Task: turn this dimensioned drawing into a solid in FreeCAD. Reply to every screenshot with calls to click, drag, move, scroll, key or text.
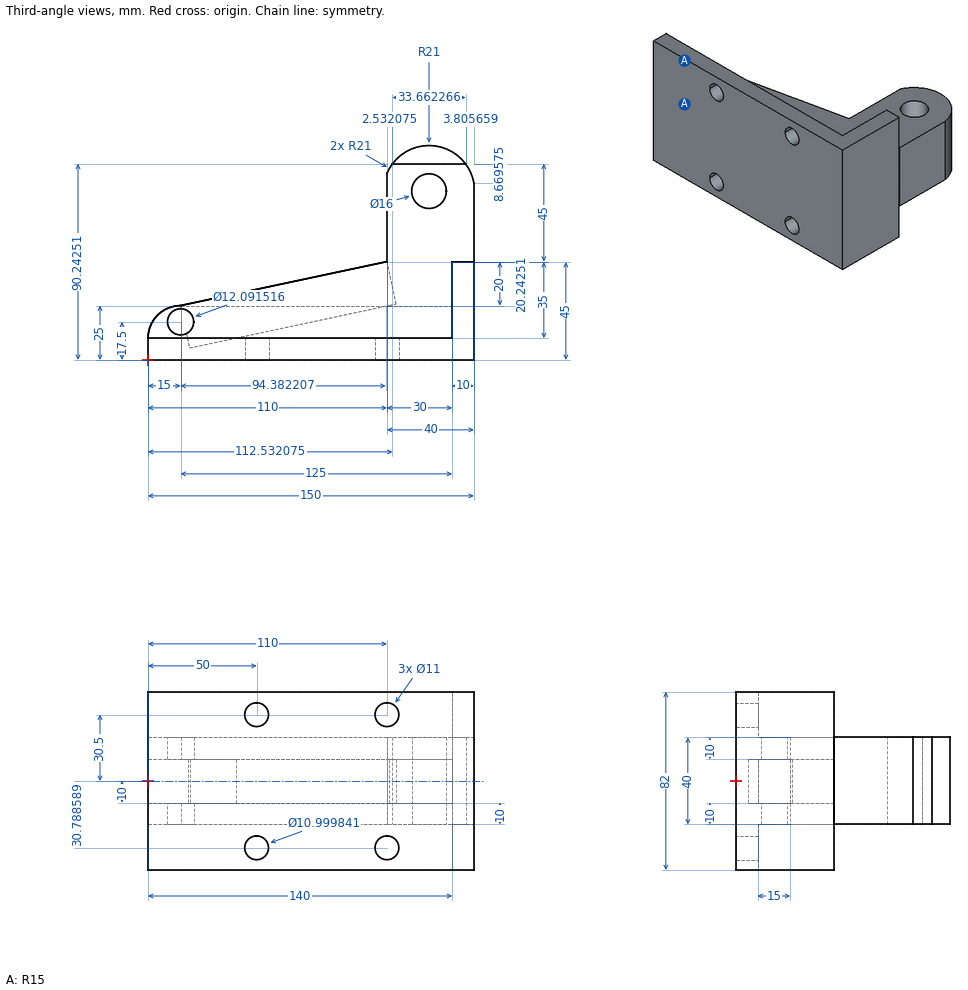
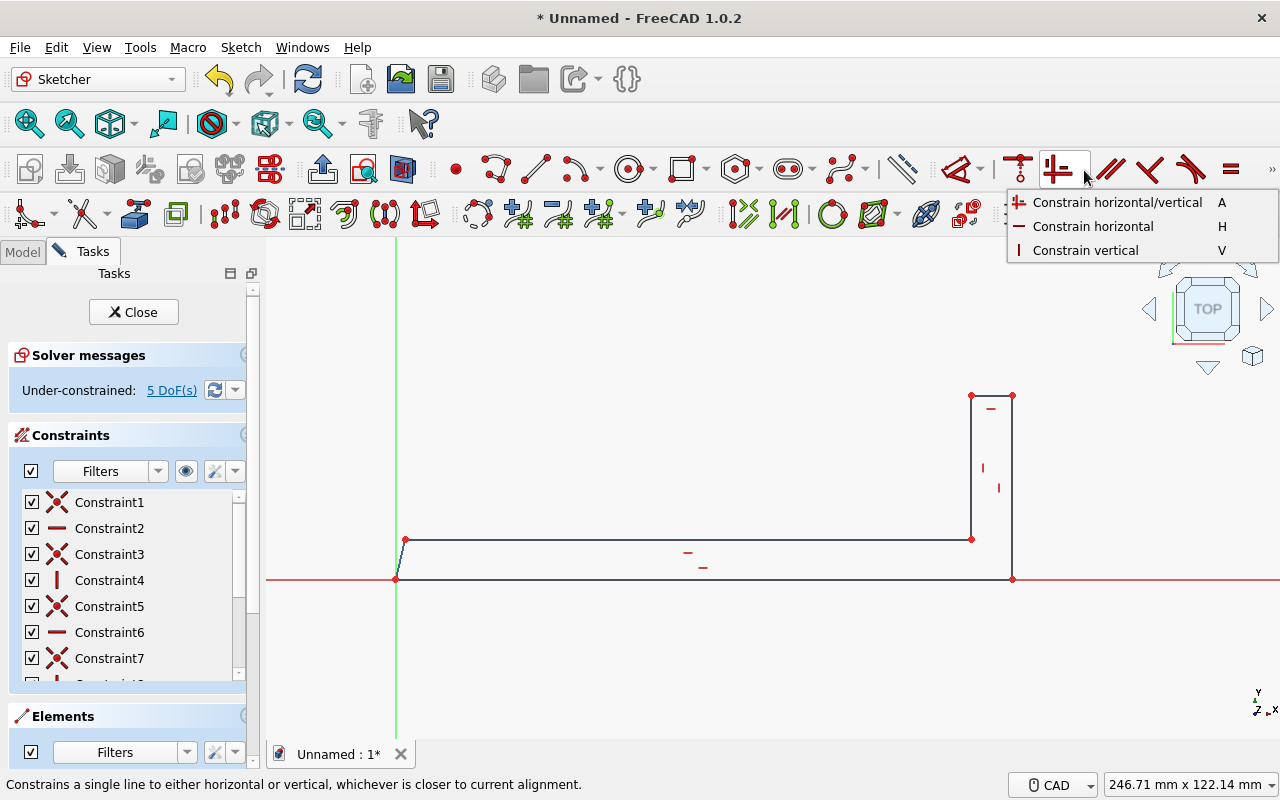
click(1143, 250)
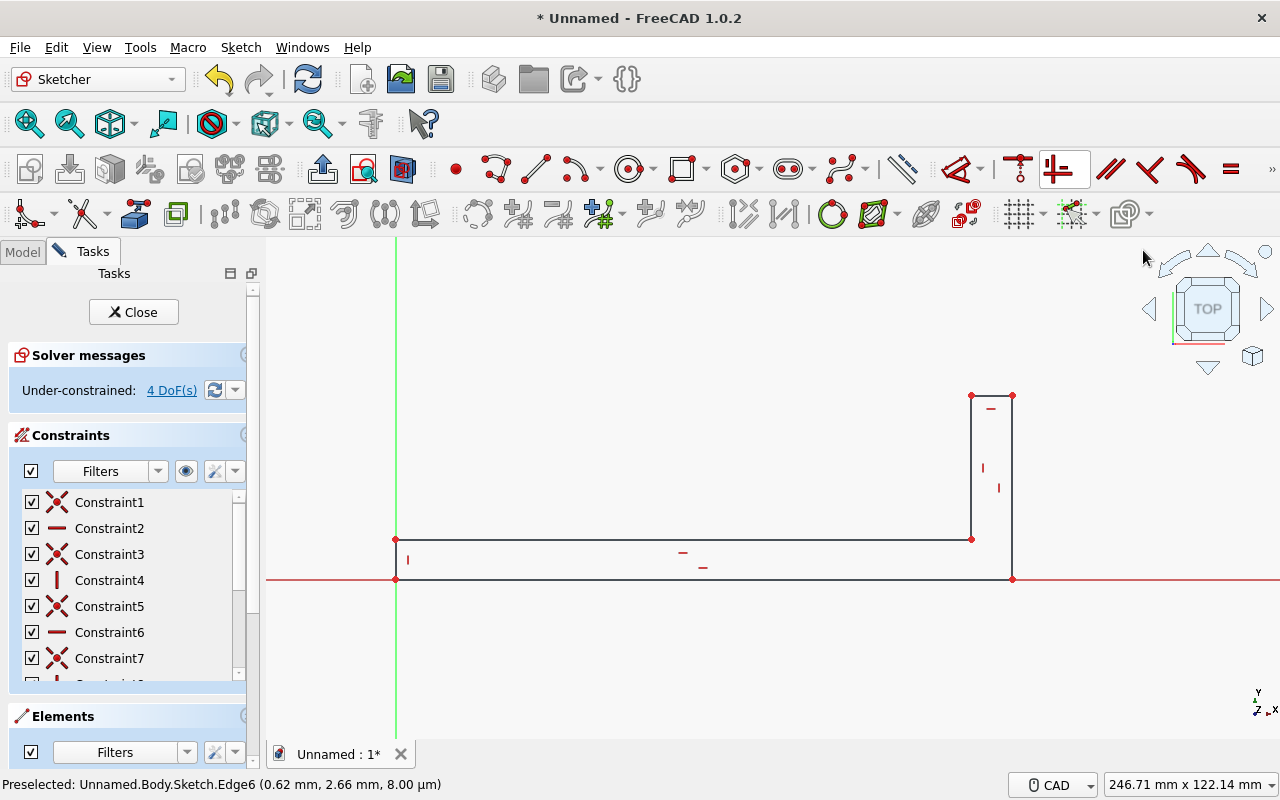
key(d)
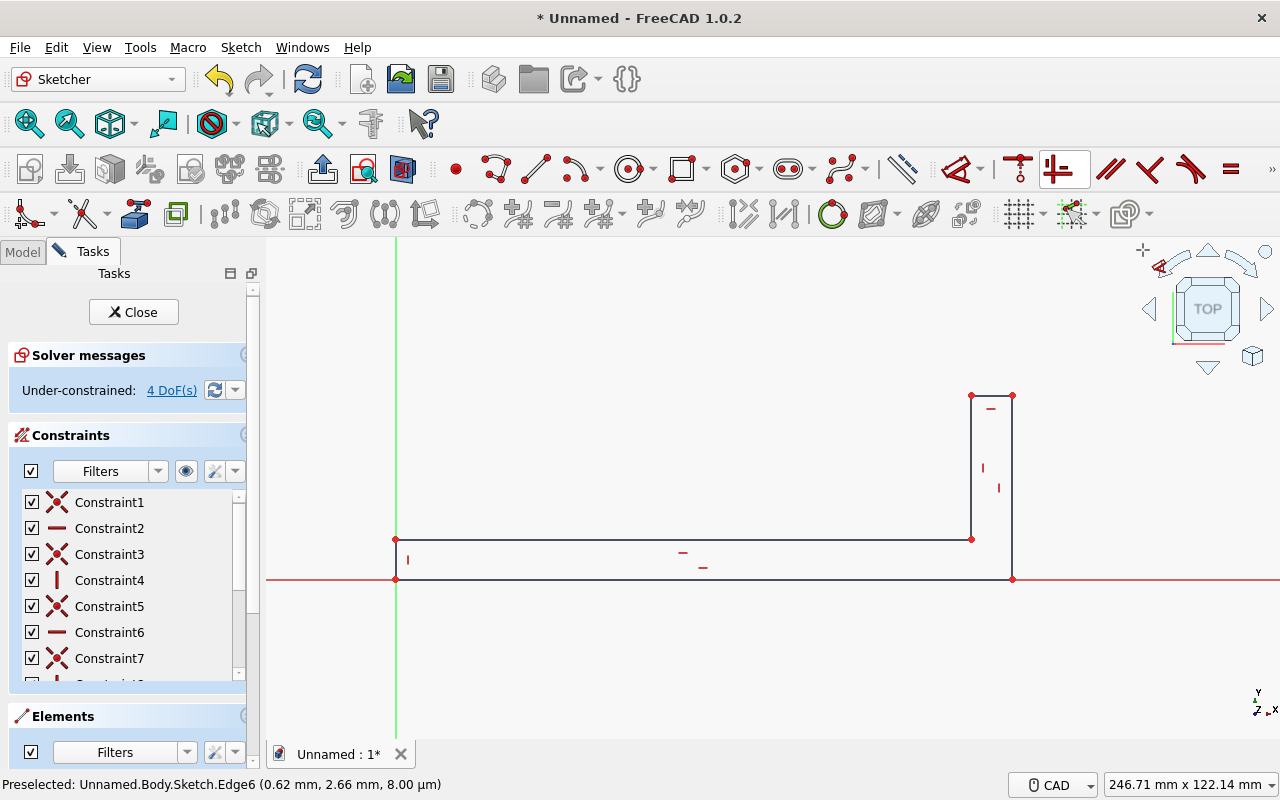
click(1012, 525)
click(1046, 488)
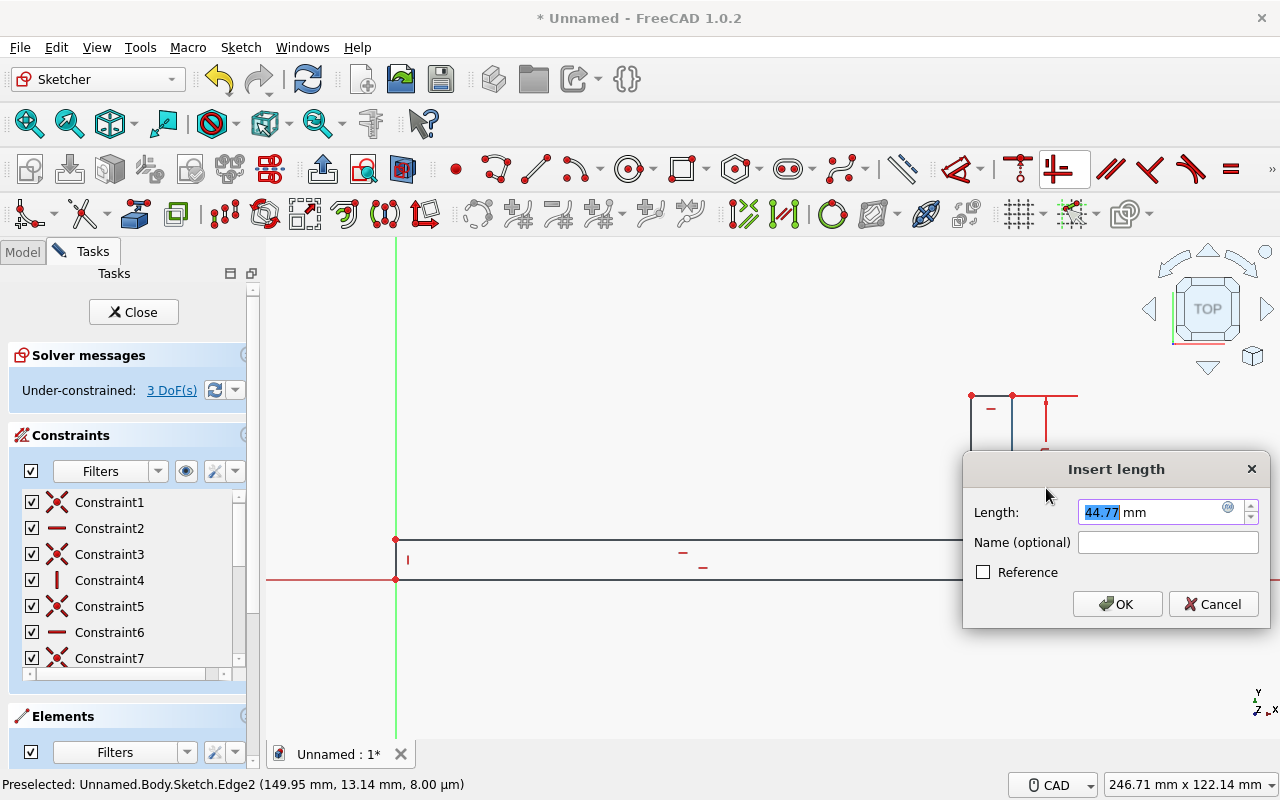
text(45)
key(Return)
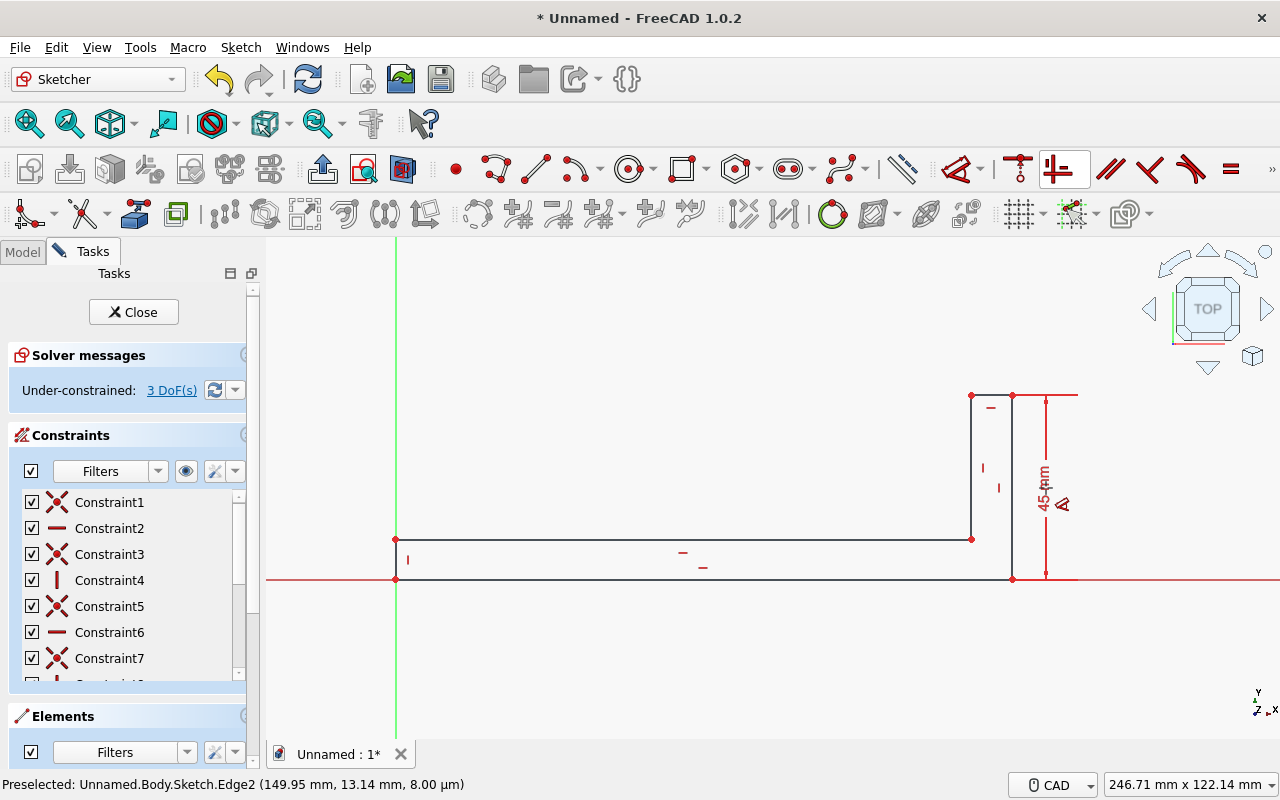
click(1000, 395)
click(992, 361)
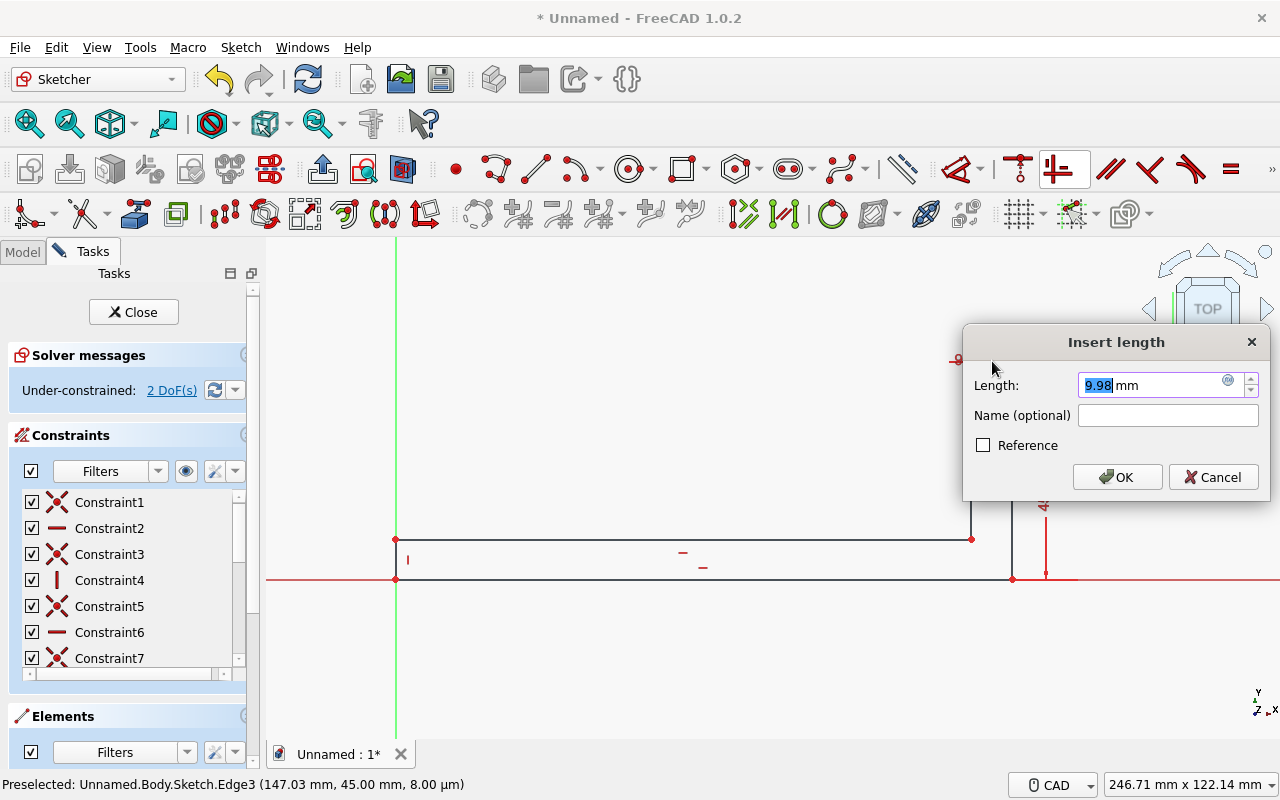
text(10)
key(Return)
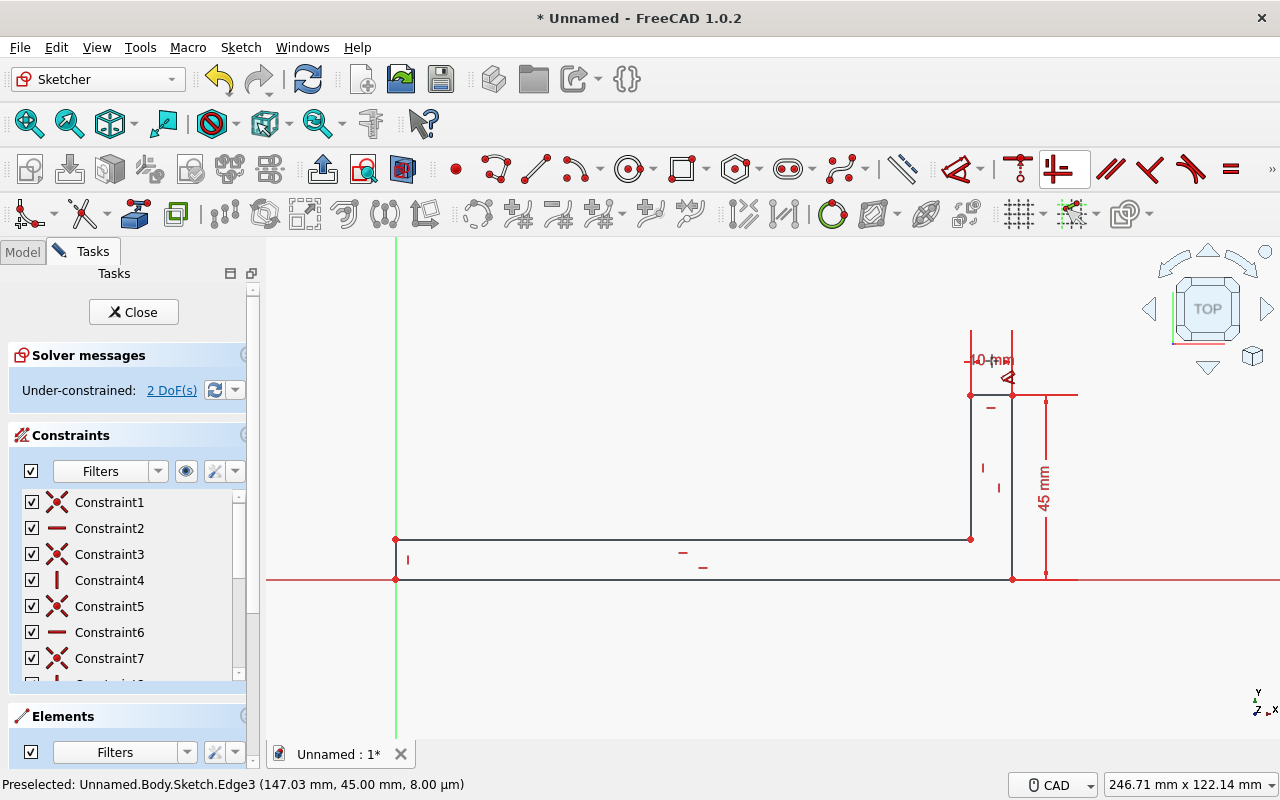
click(971, 439)
click(937, 468)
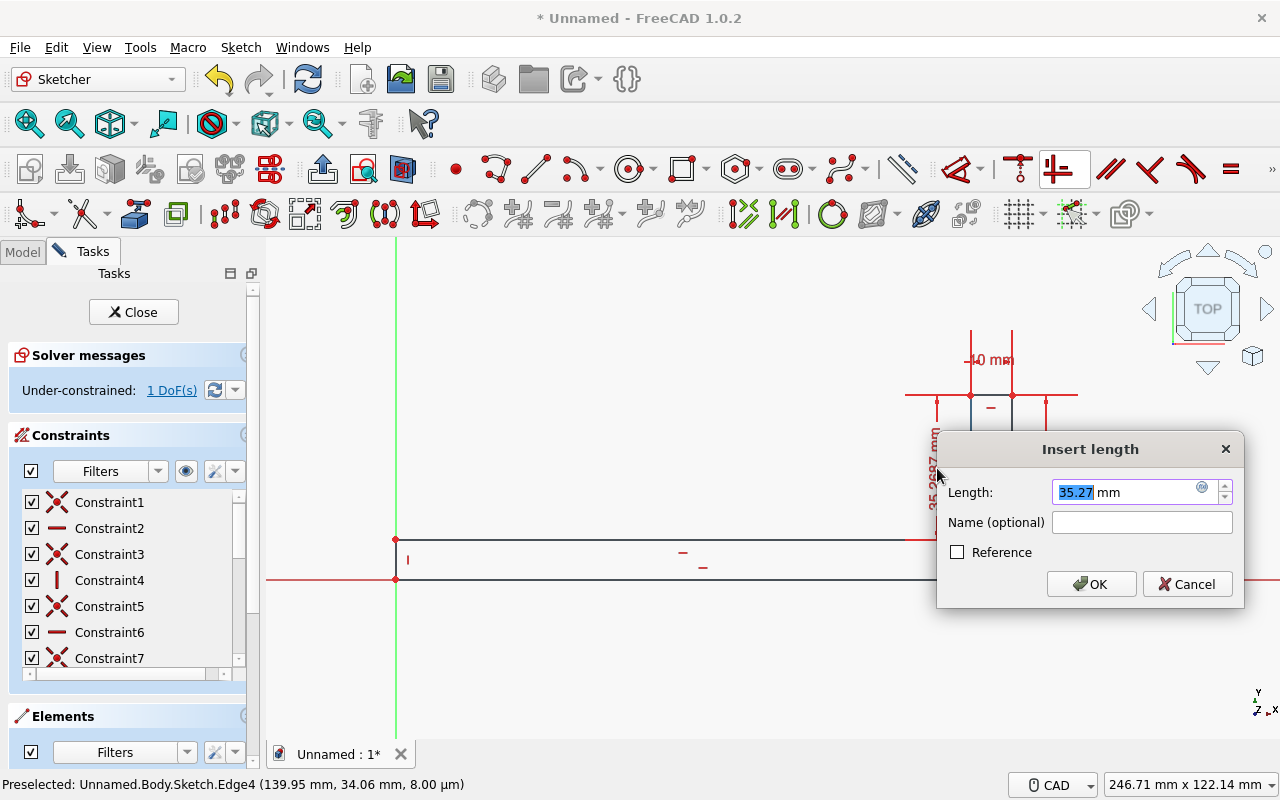
text(35)
key(Return)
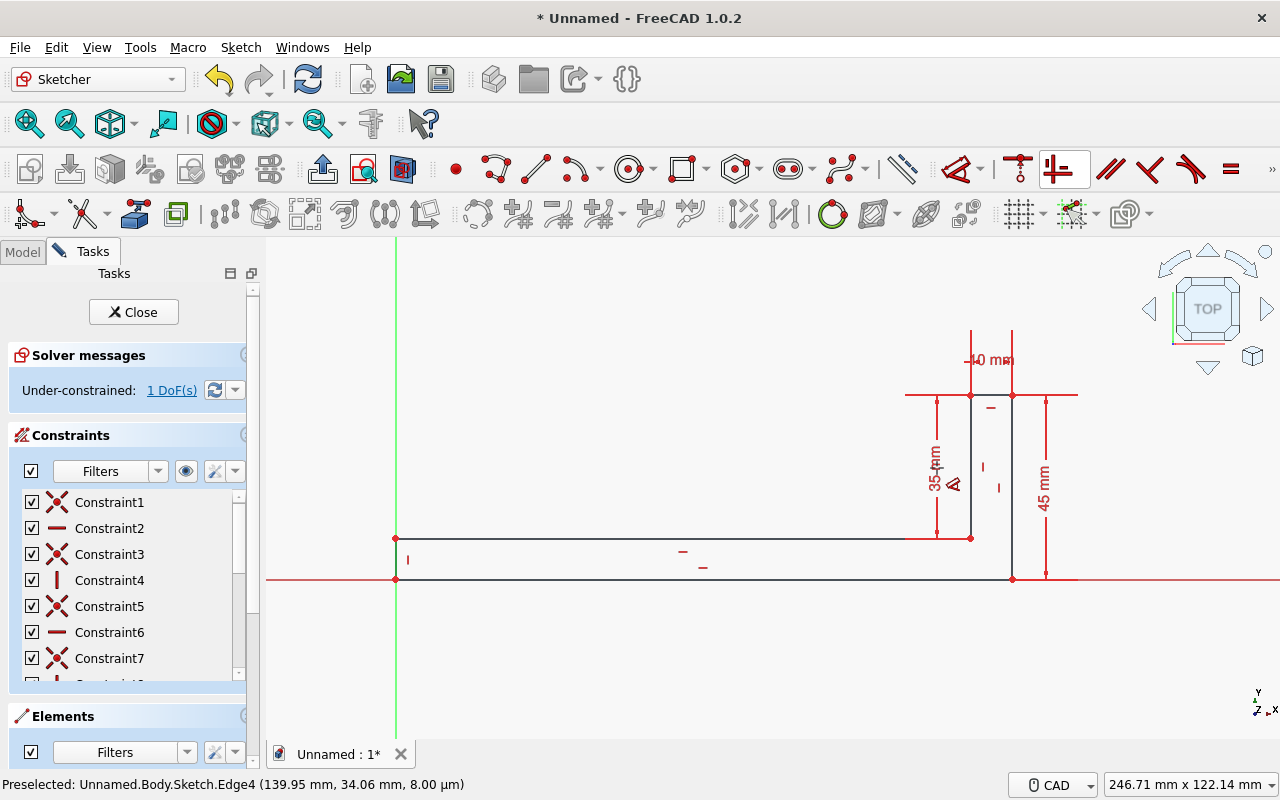
click(581, 580)
click(704, 614)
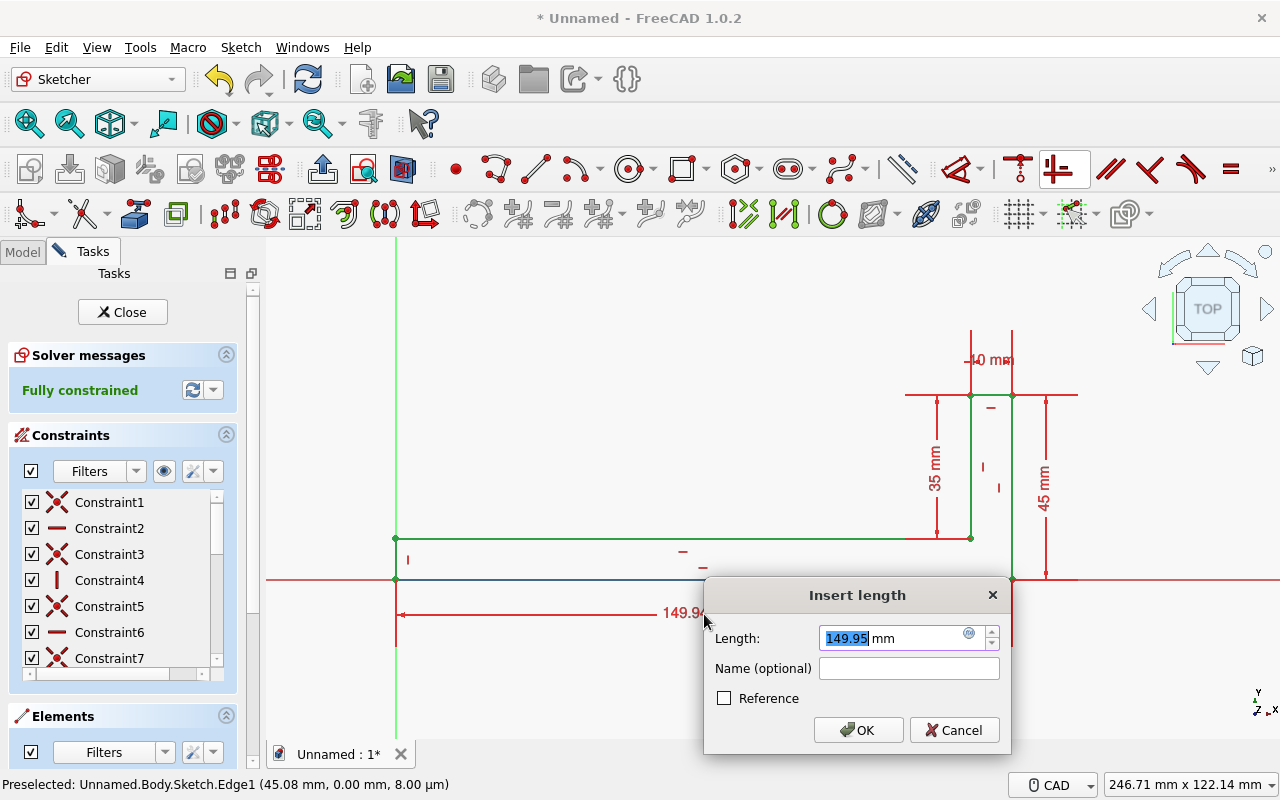
text(150)
key(Return)
key(Escape)